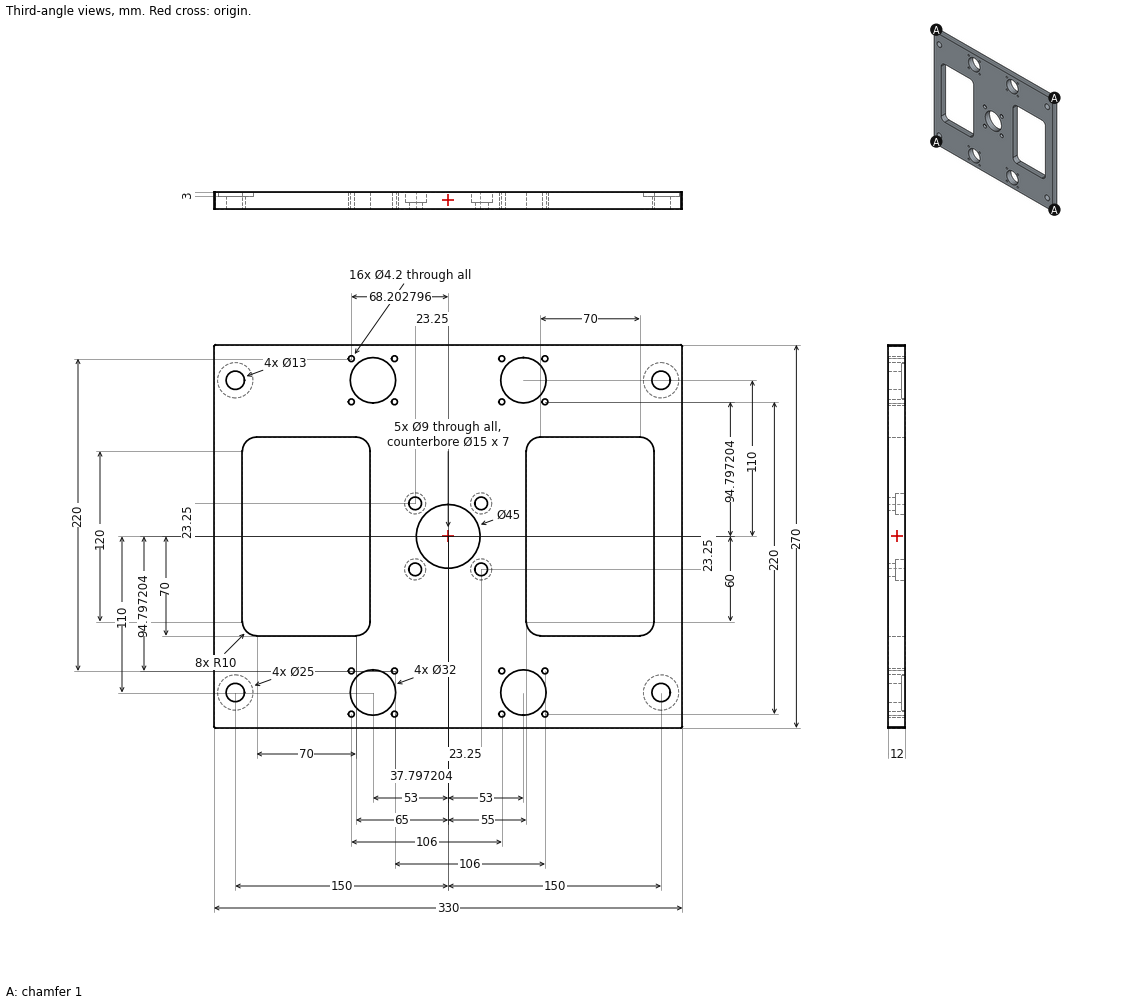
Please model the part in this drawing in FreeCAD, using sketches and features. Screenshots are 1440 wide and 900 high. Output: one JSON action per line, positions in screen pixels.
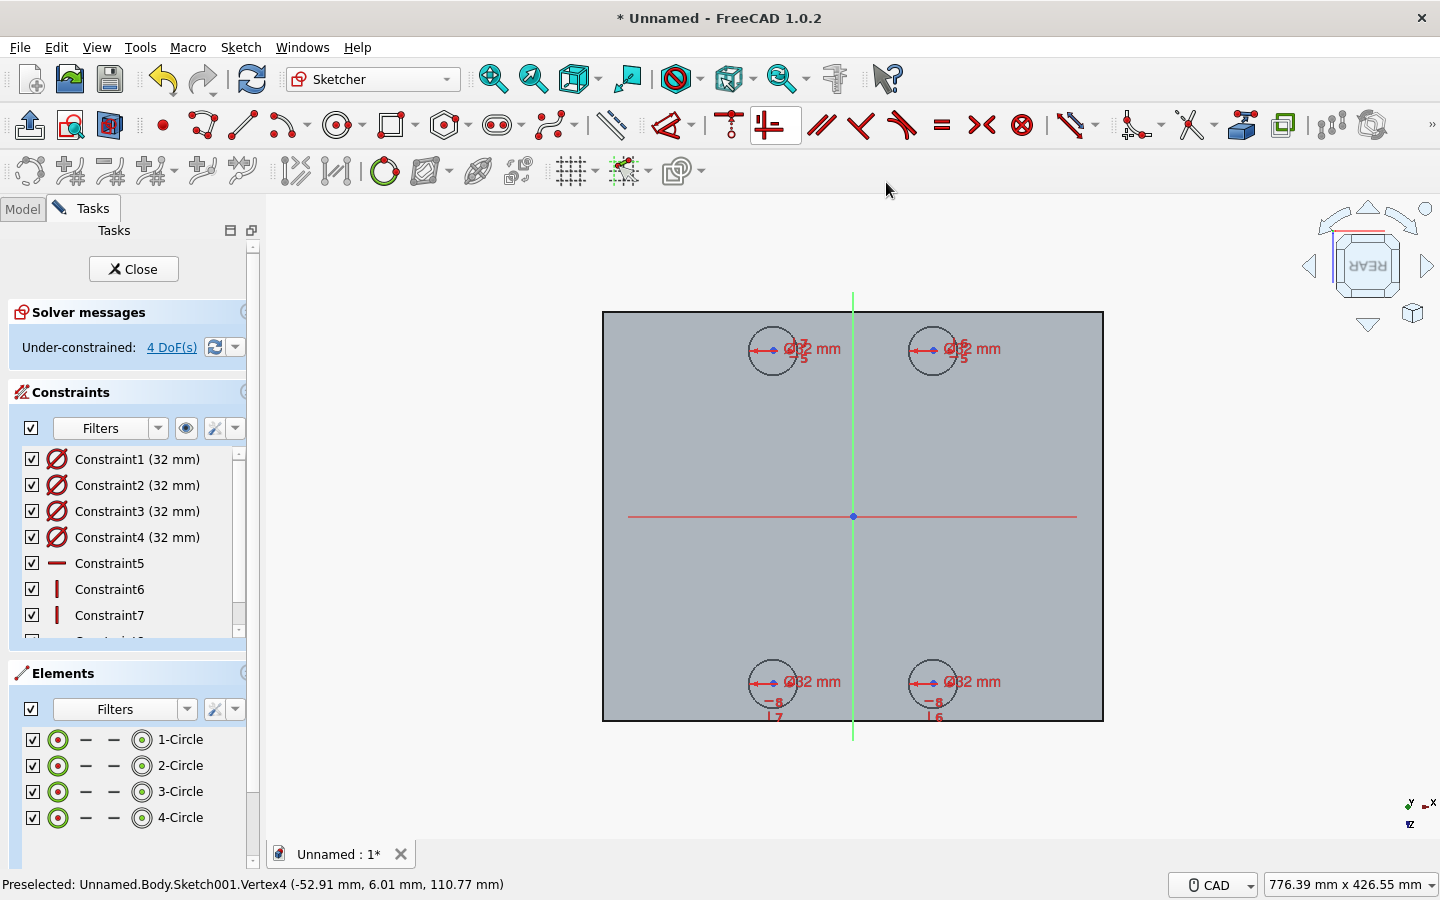
{"action": "left_click", "coordinate": [773, 351]}
{"action": "left_click", "coordinate": [813, 317]}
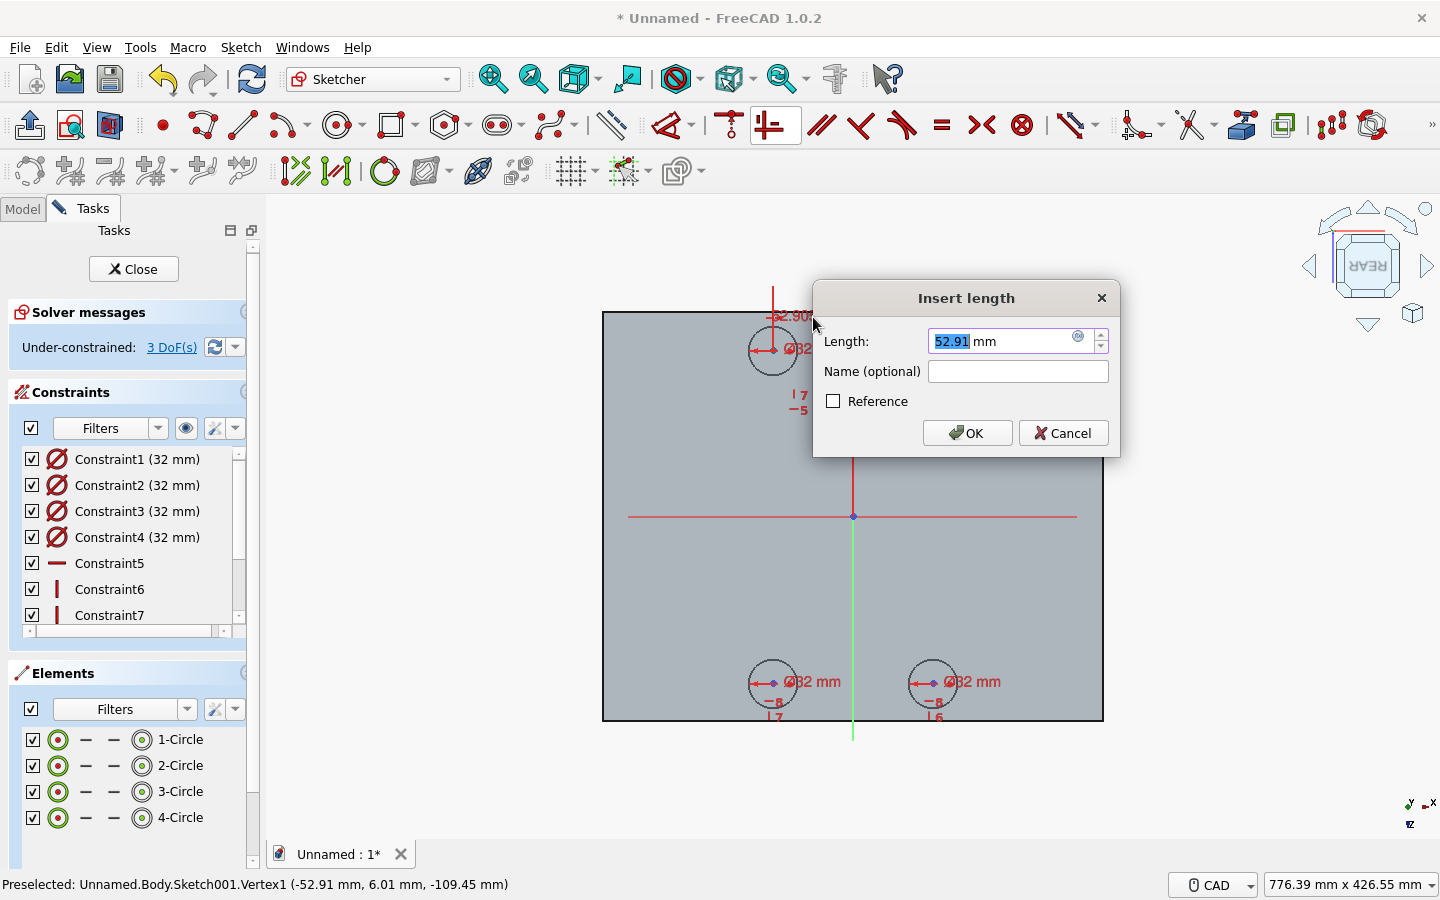
{"action": "type", "text": "53"}
{"action": "key", "text": "Return"}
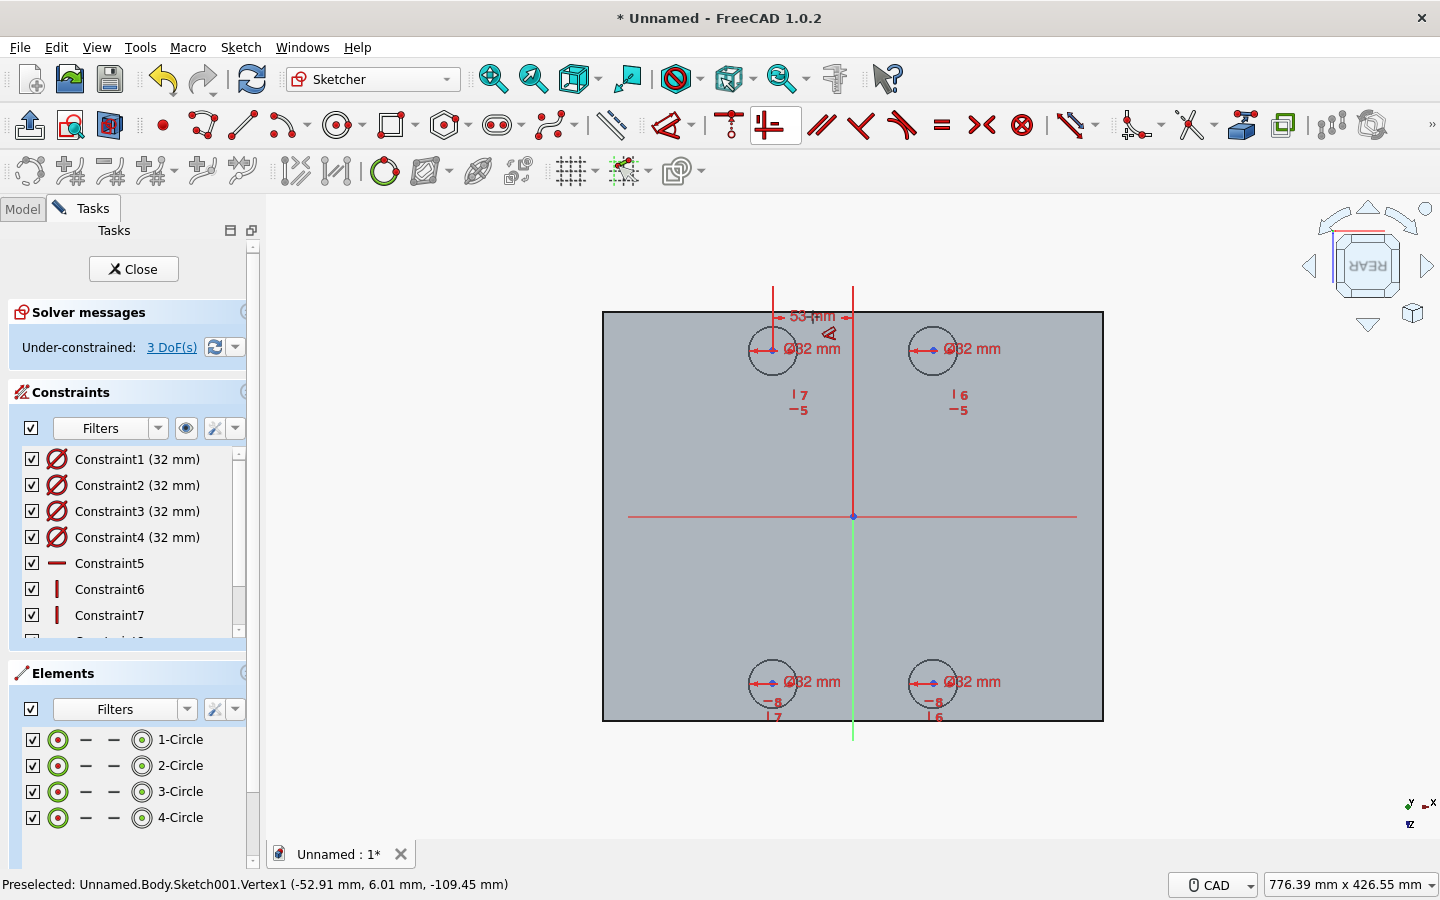
{"action": "left_click", "coordinate": [933, 351]}
{"action": "left_click", "coordinate": [893, 317]}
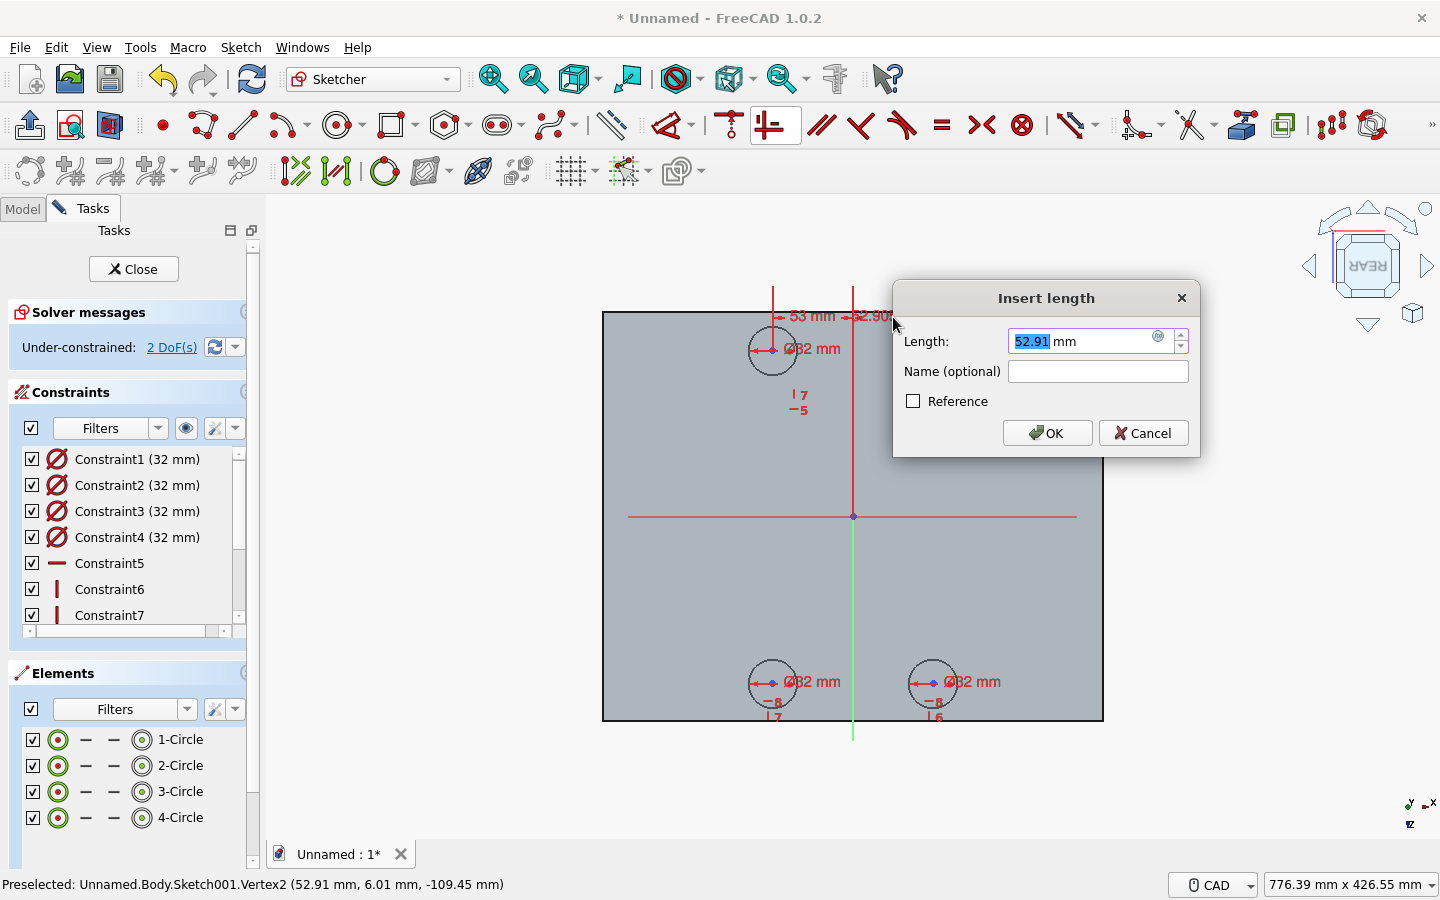
{"action": "type", "text": "53"}
{"action": "key", "text": "Return"}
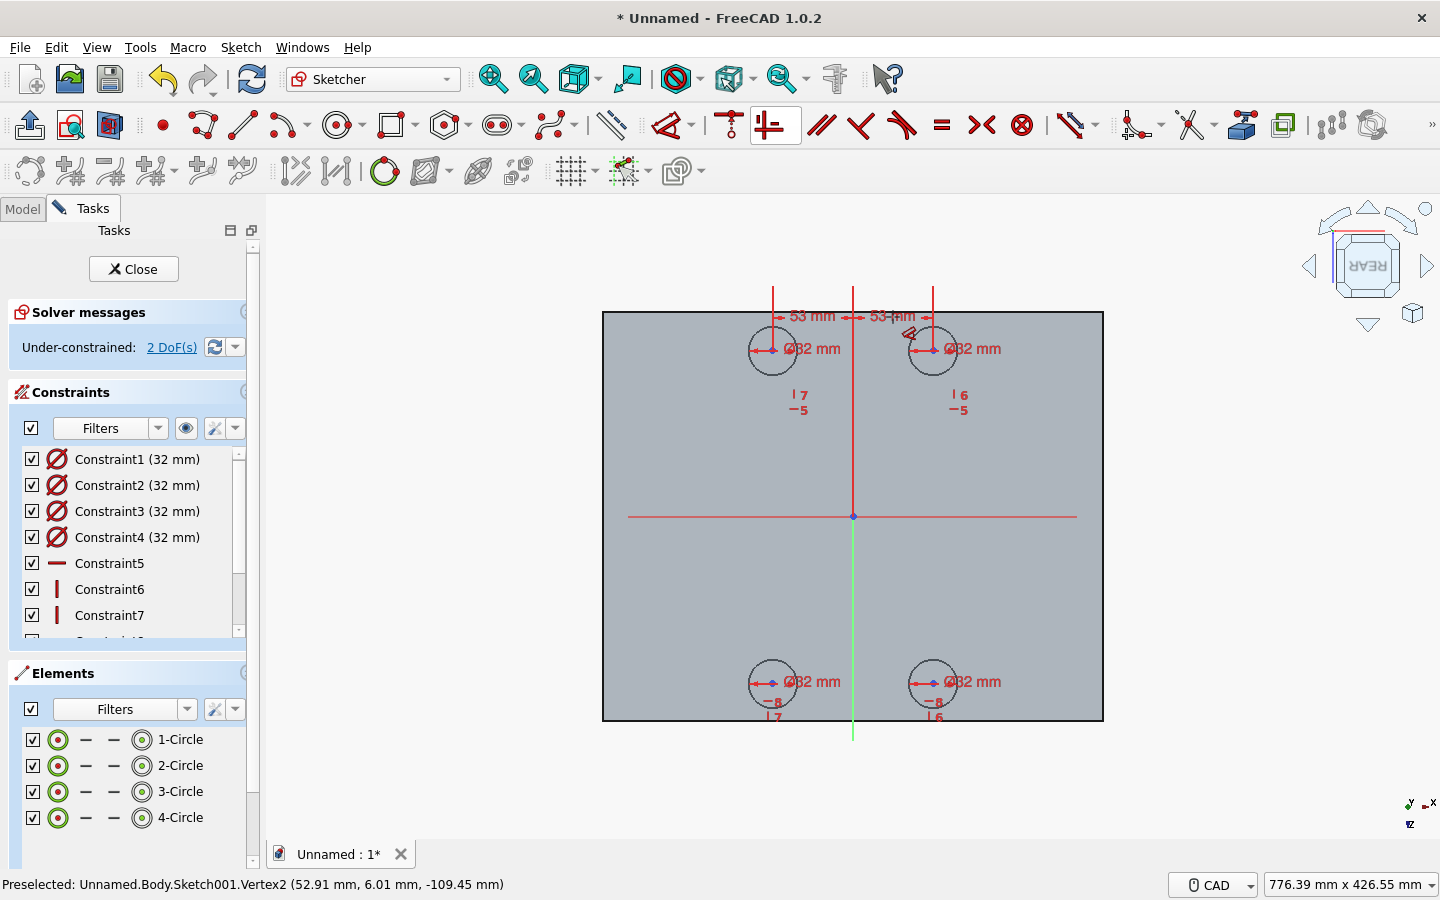
{"action": "left_click", "coordinate": [773, 351]}
{"action": "left_click", "coordinate": [739, 434]}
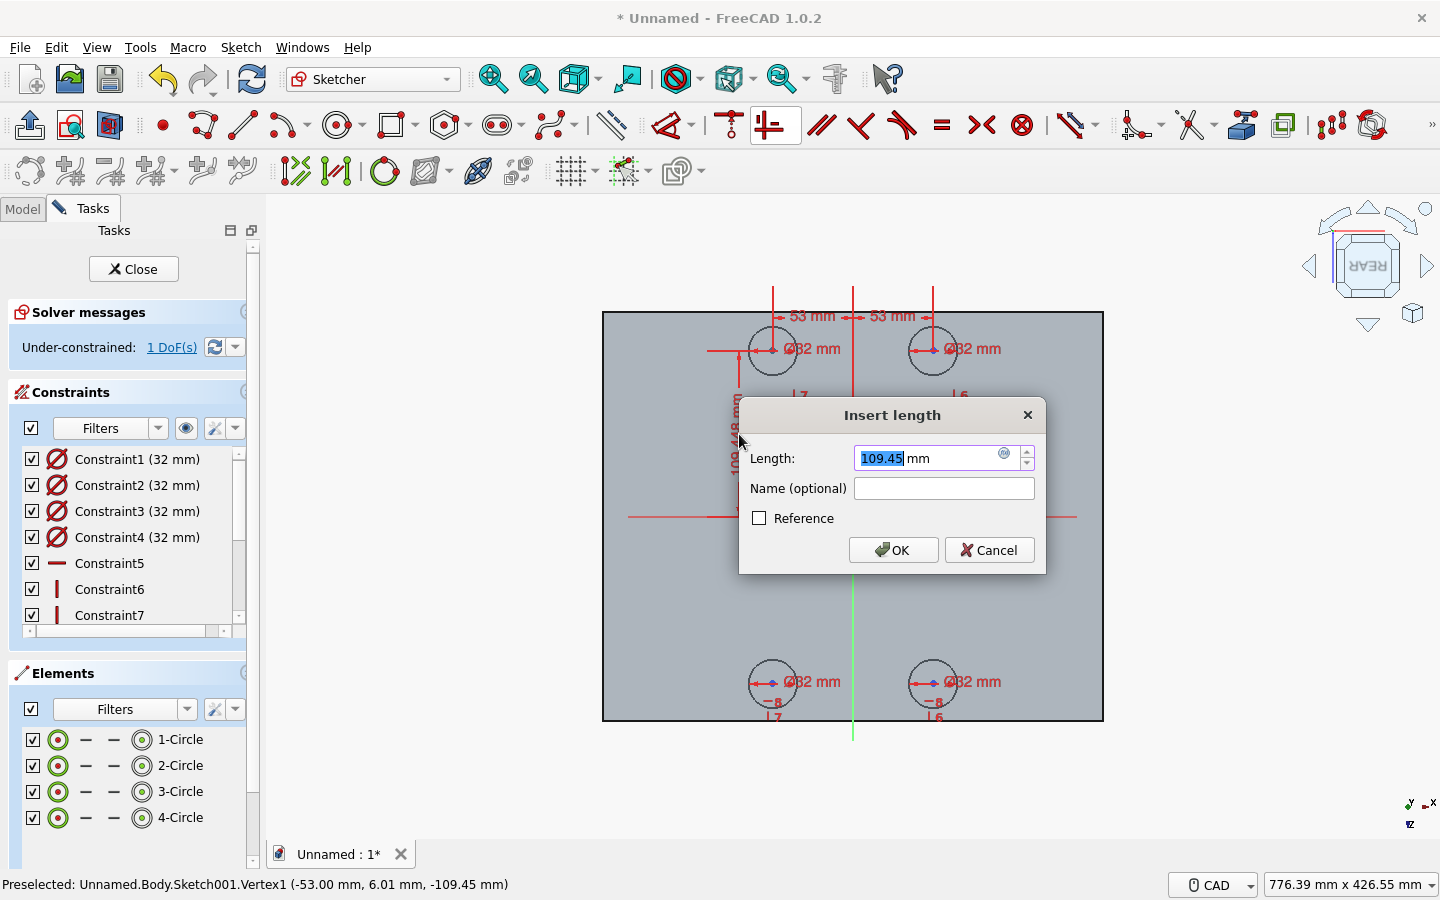
{"action": "type", "text": "110"}
{"action": "key", "text": "Return"}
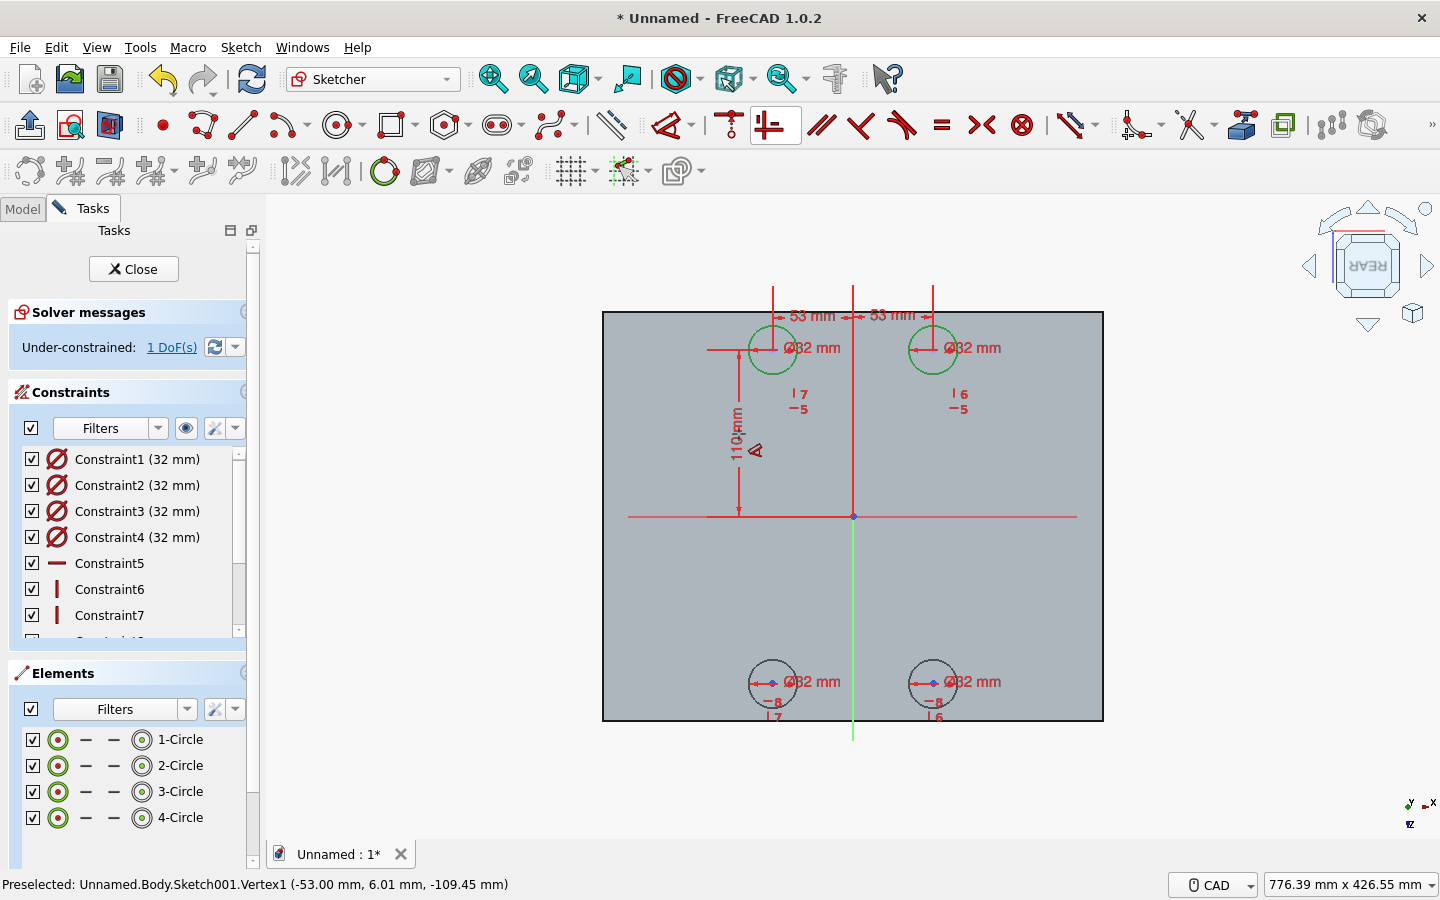
{"action": "left_click", "coordinate": [933, 684]}
{"action": "left_click", "coordinate": [967, 600]}